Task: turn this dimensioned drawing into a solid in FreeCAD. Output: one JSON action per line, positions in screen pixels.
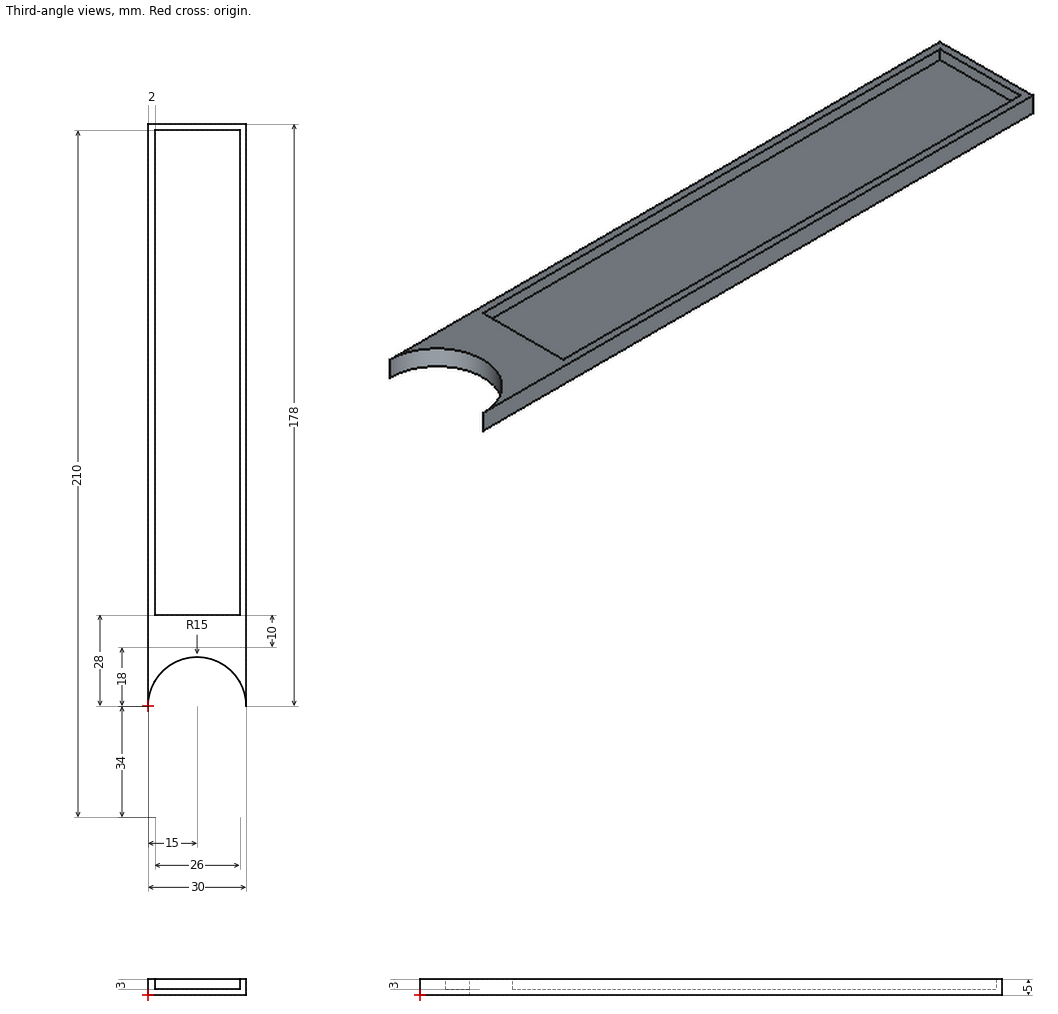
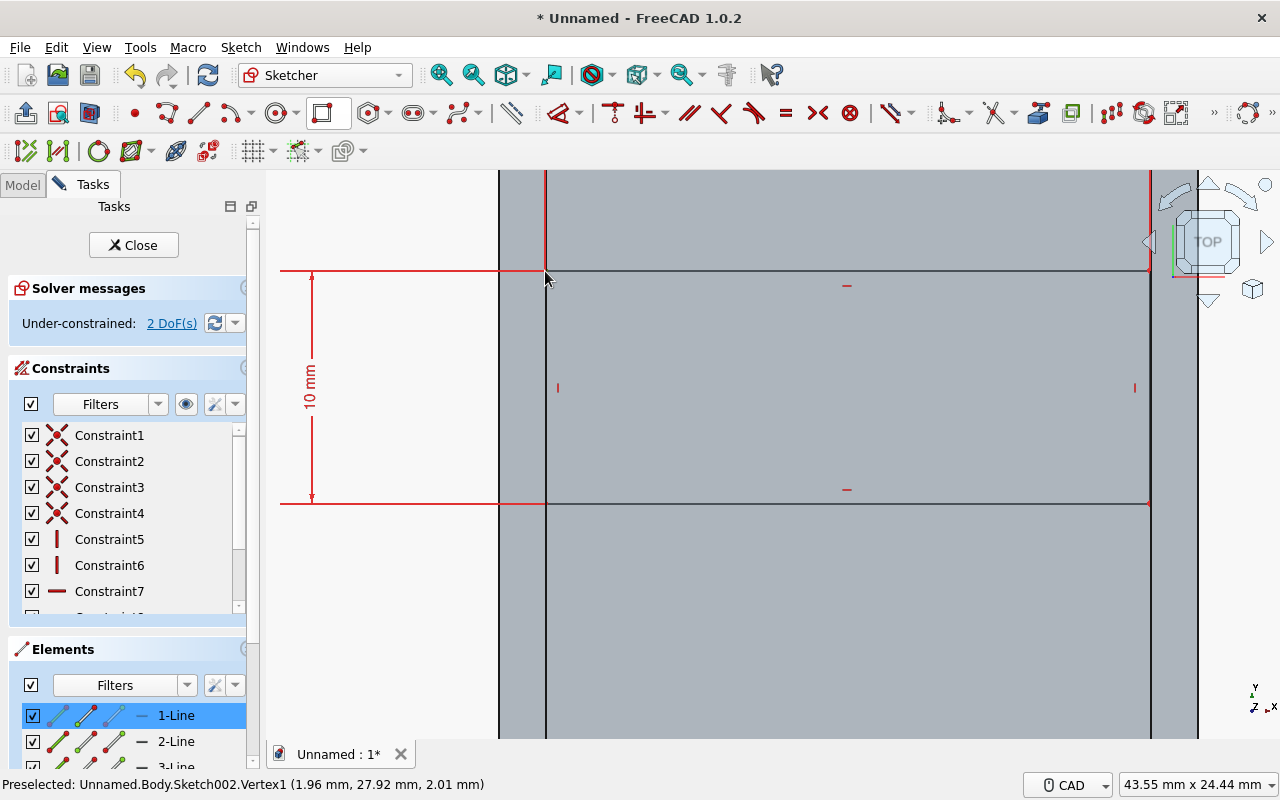
{"action": "key", "text": "l"}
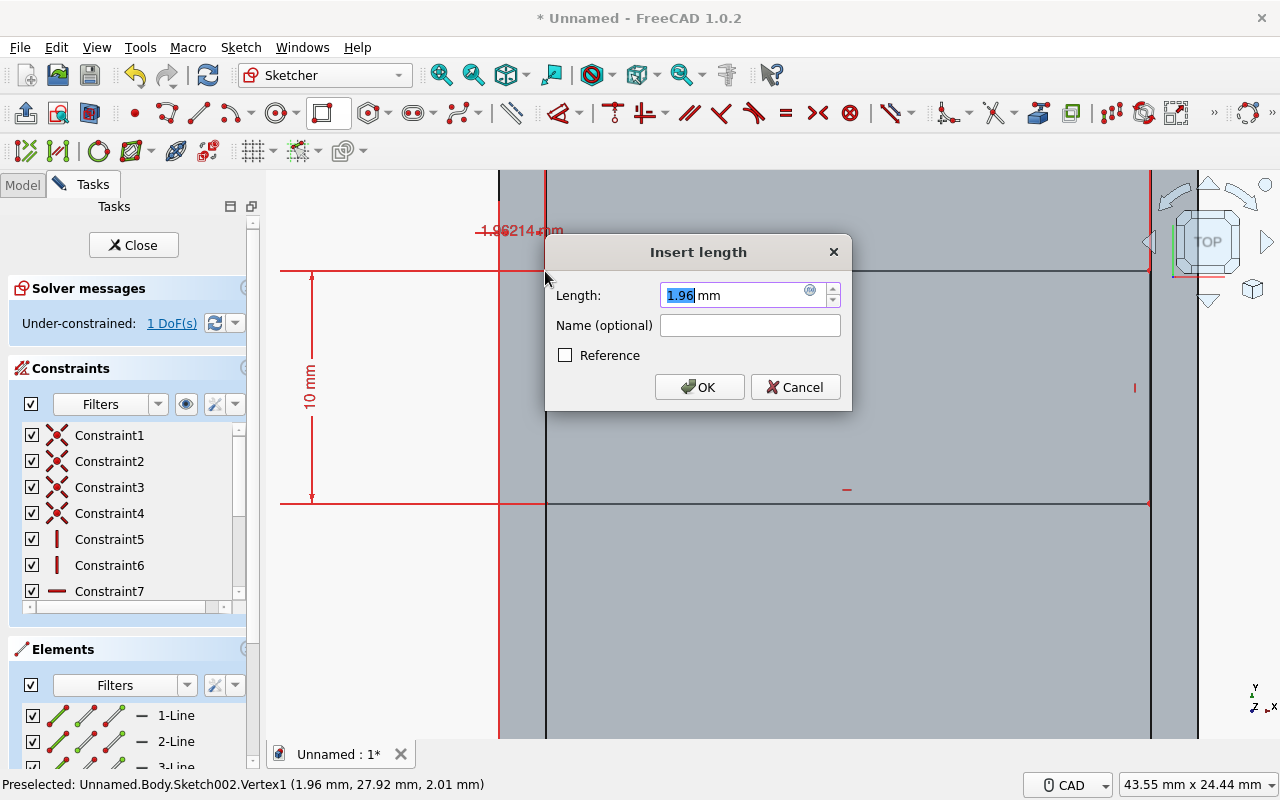
{"action": "type", "text": "2"}
{"action": "key", "text": "Return"}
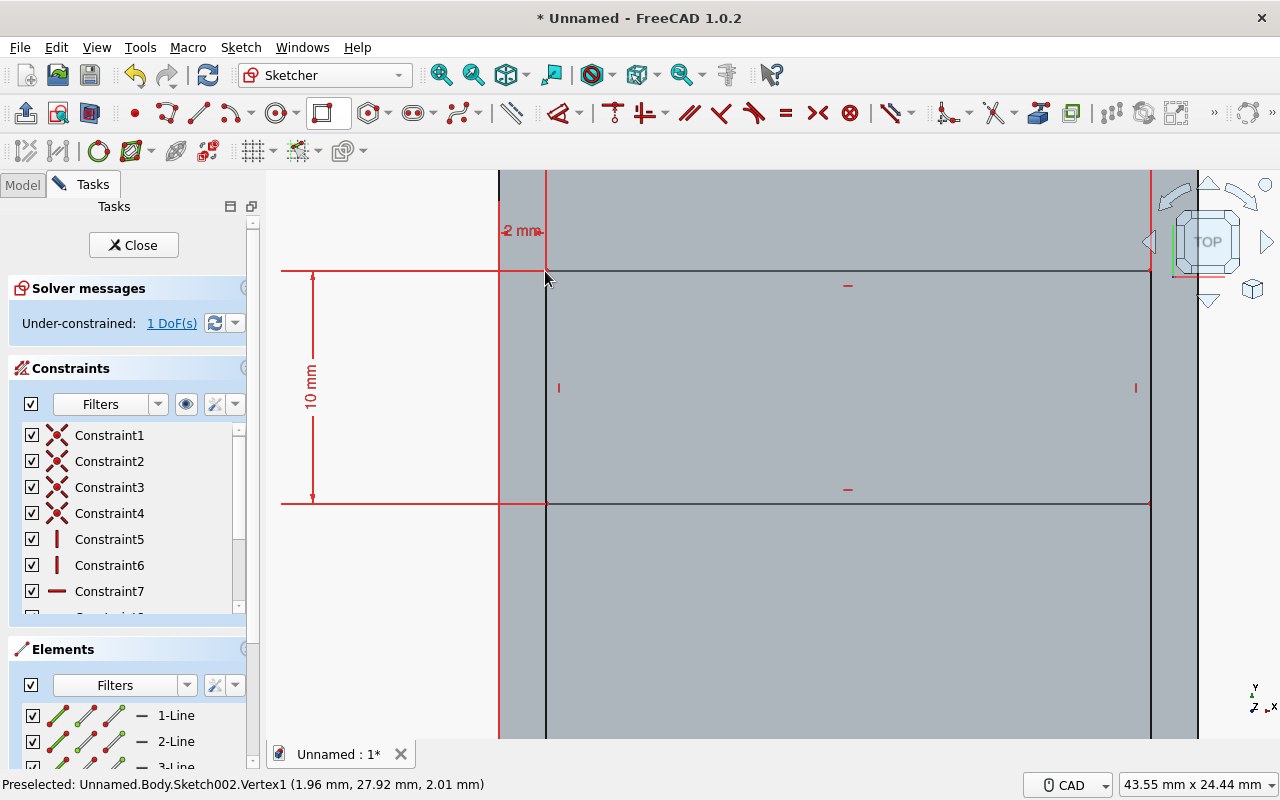
{"action": "left_click", "coordinate": [546, 271]}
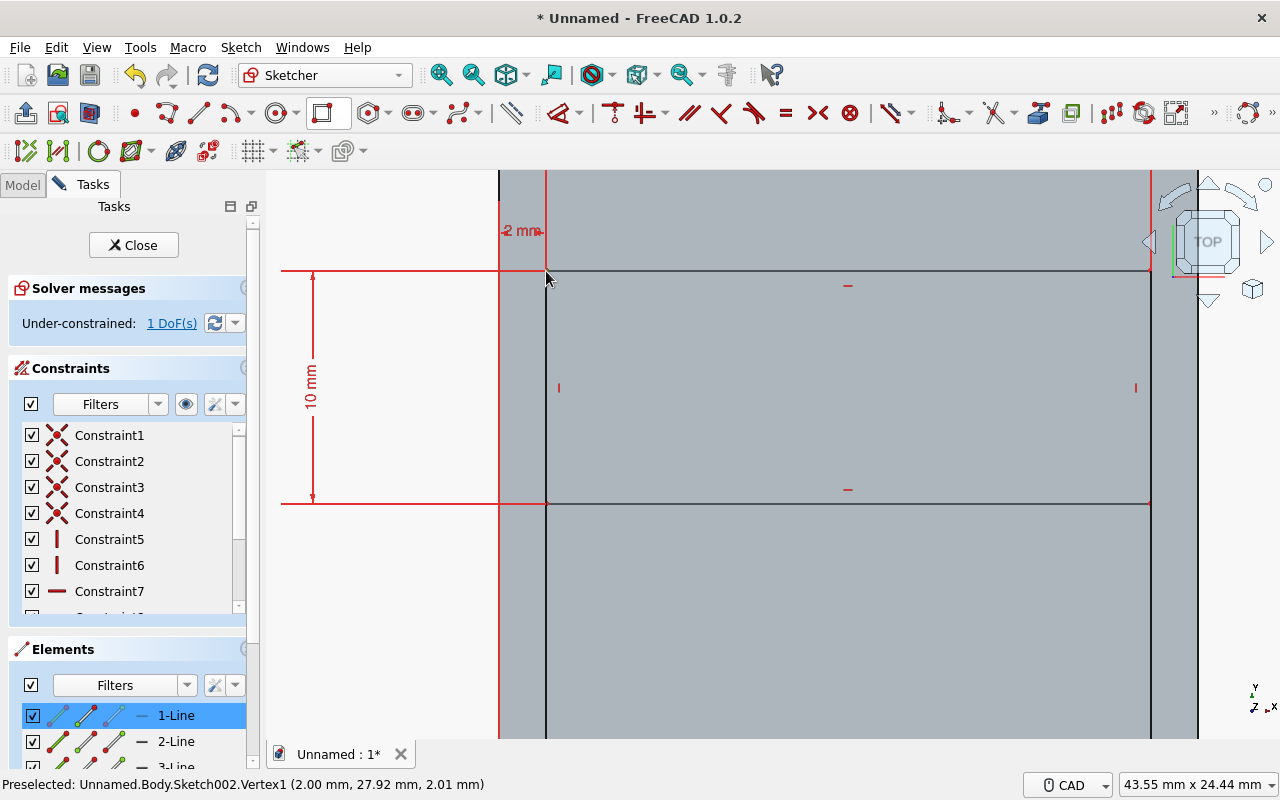
{"action": "key", "text": "i"}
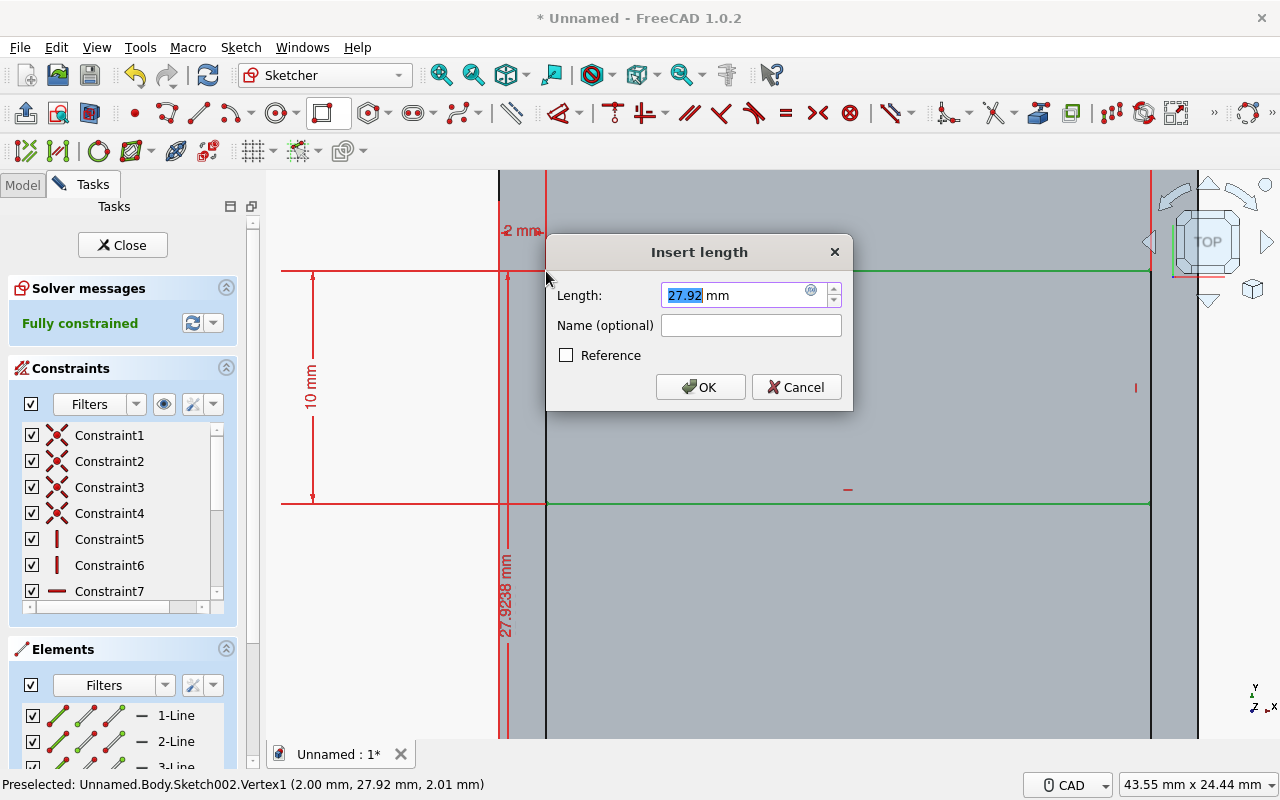
{"action": "type", "text": "28"}
{"action": "key", "text": "Return"}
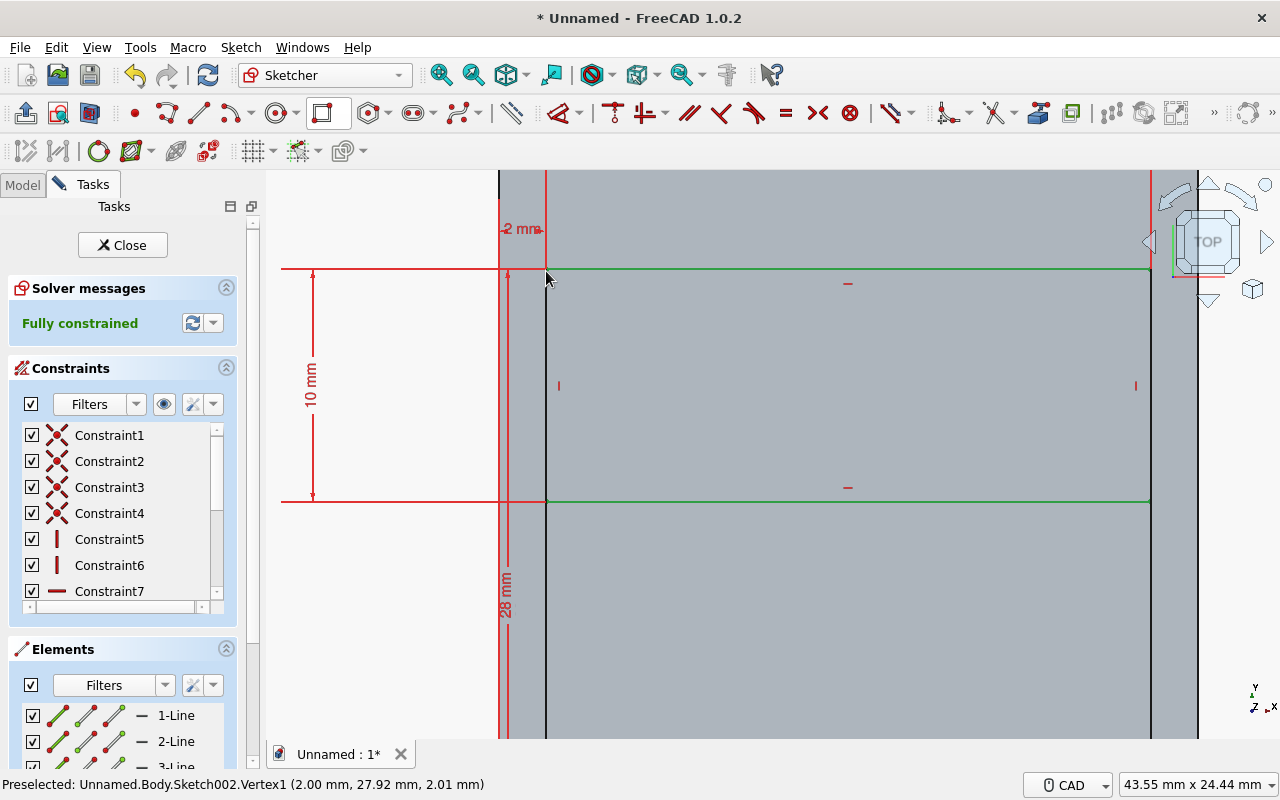
{"action": "left_click", "coordinate": [123, 245]}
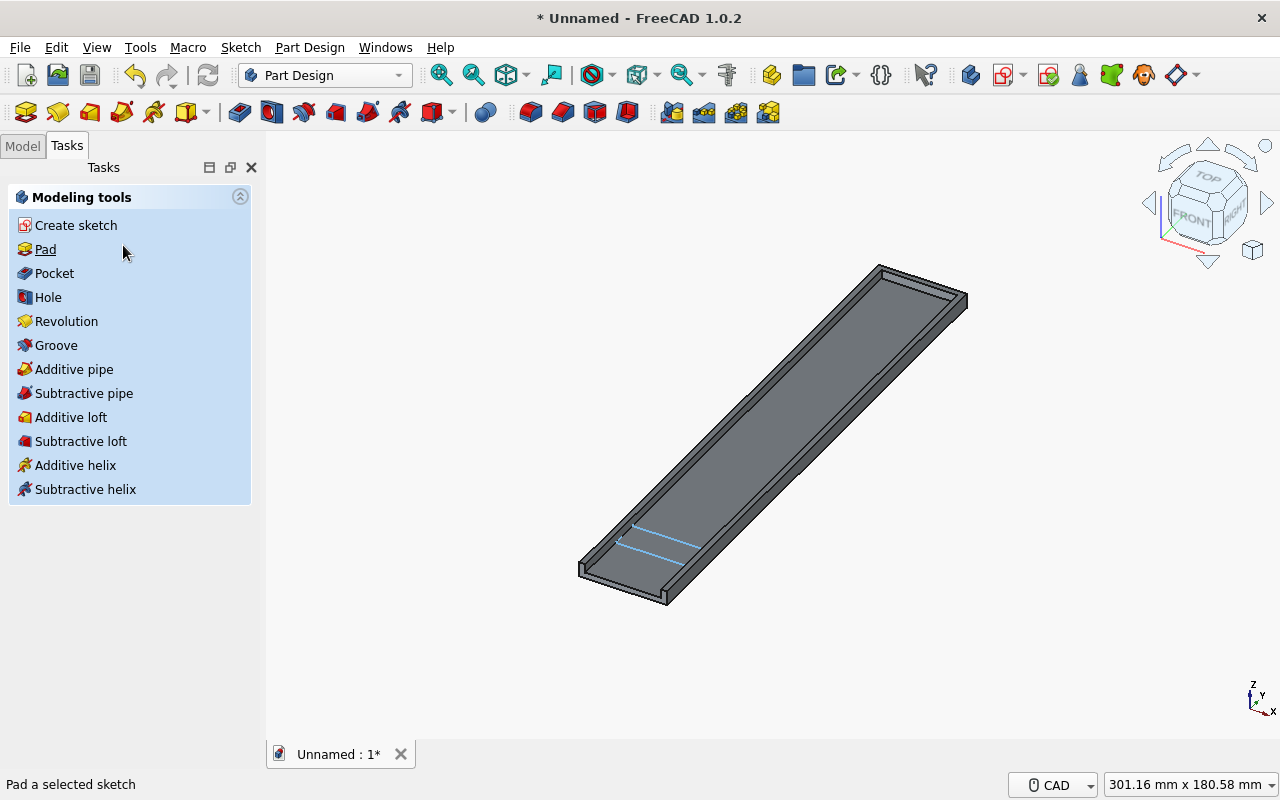
{"action": "left_click", "coordinate": [26, 112]}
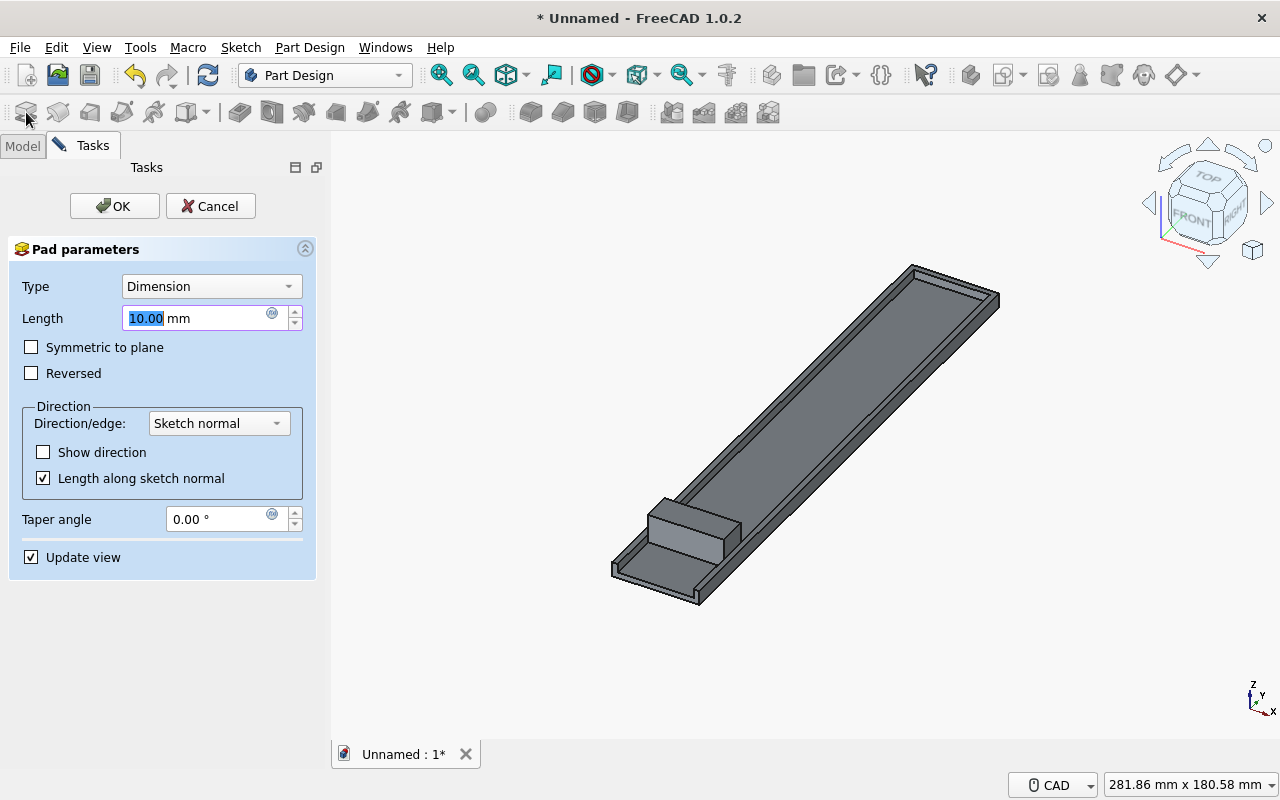
{"action": "type", "text": "3"}
{"action": "key", "text": "Tab"}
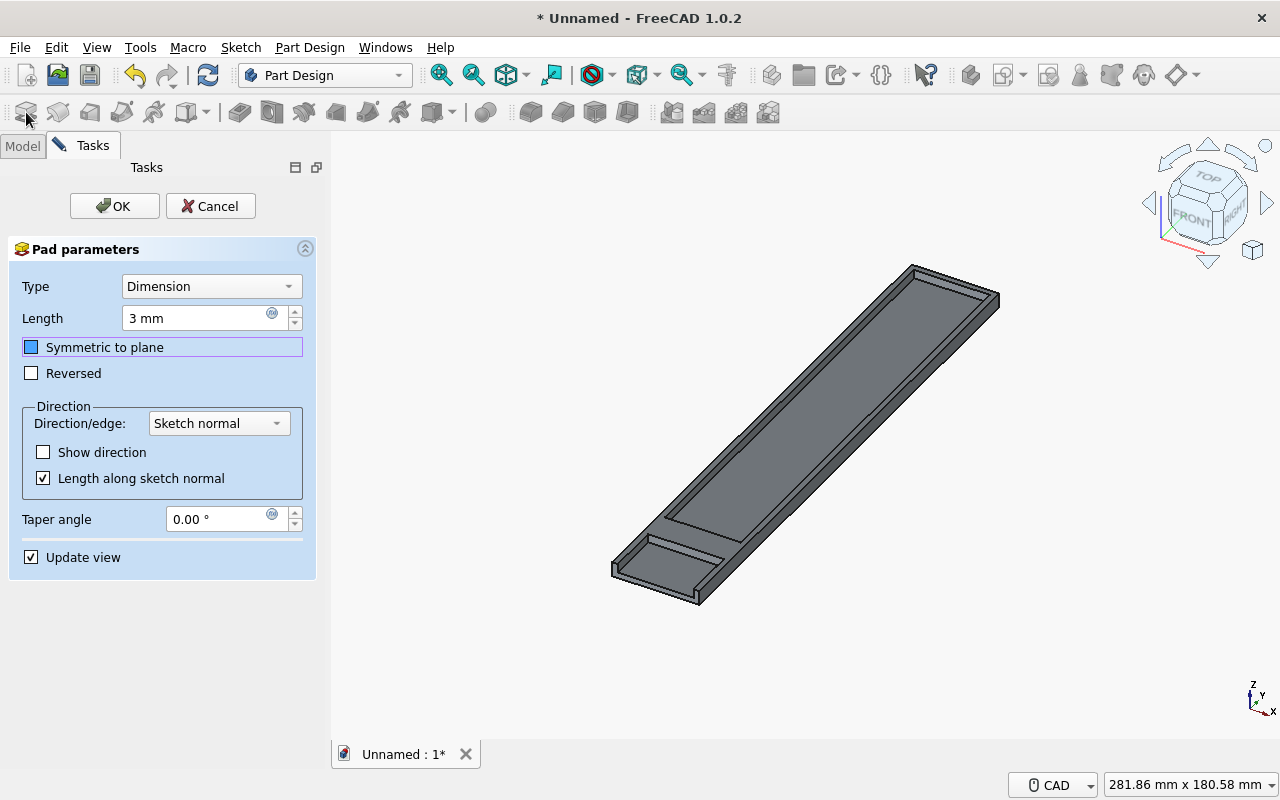
{"action": "left_click", "coordinate": [115, 206]}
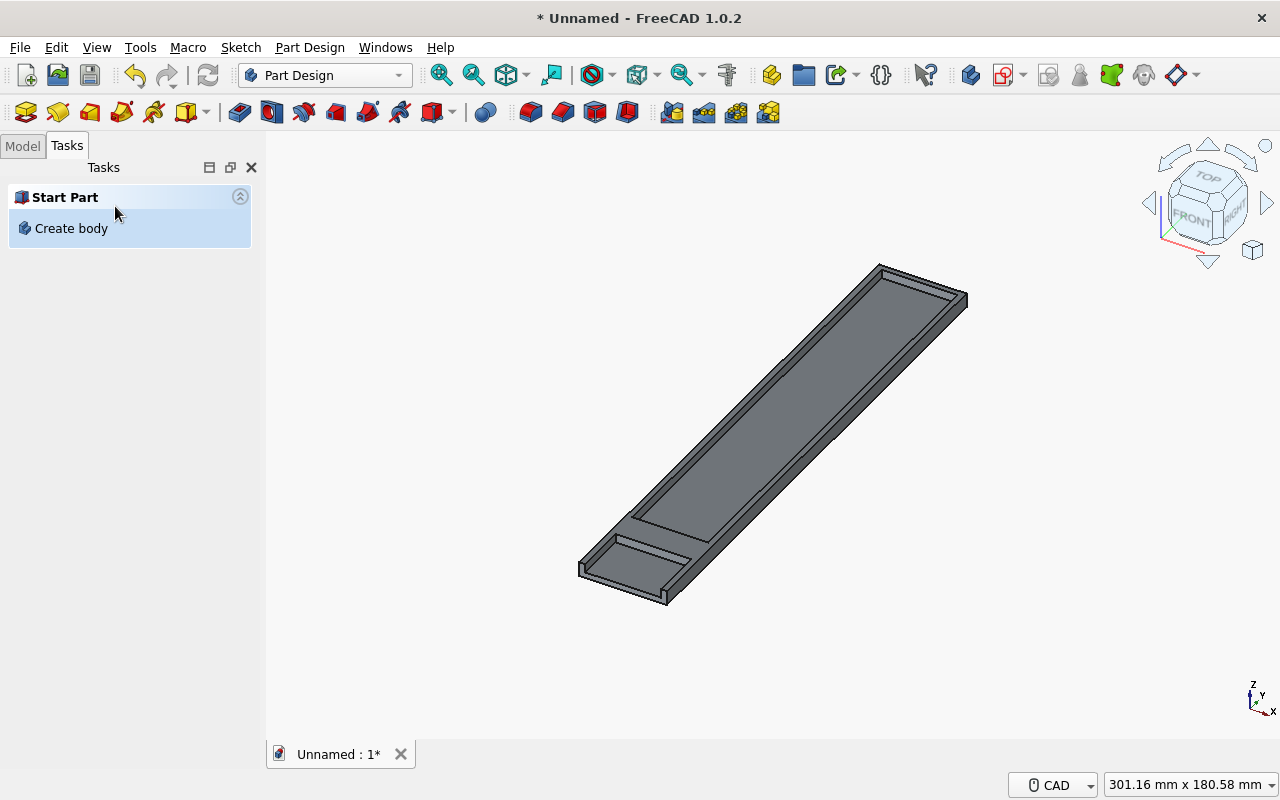
{"action": "left_click", "coordinate": [866, 343]}